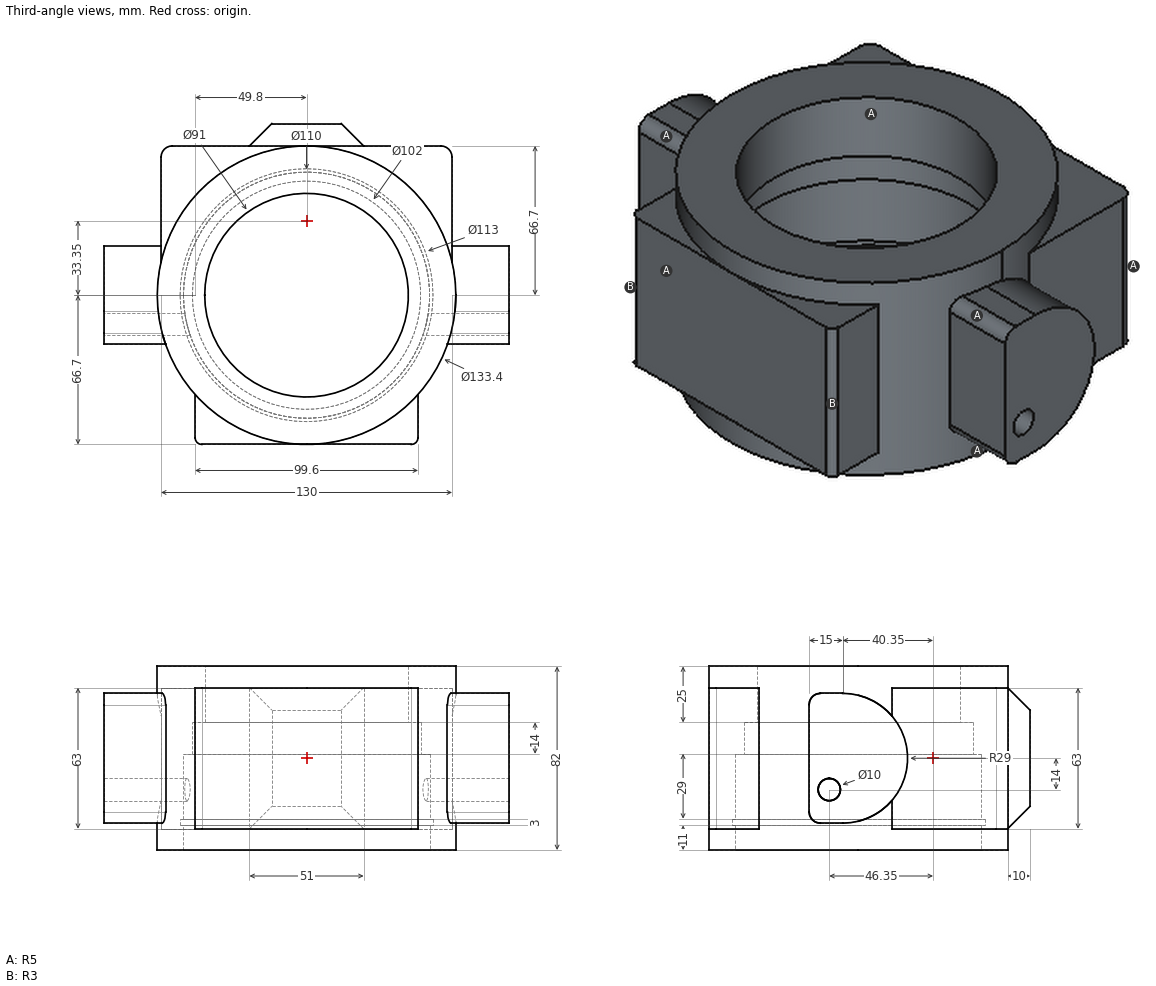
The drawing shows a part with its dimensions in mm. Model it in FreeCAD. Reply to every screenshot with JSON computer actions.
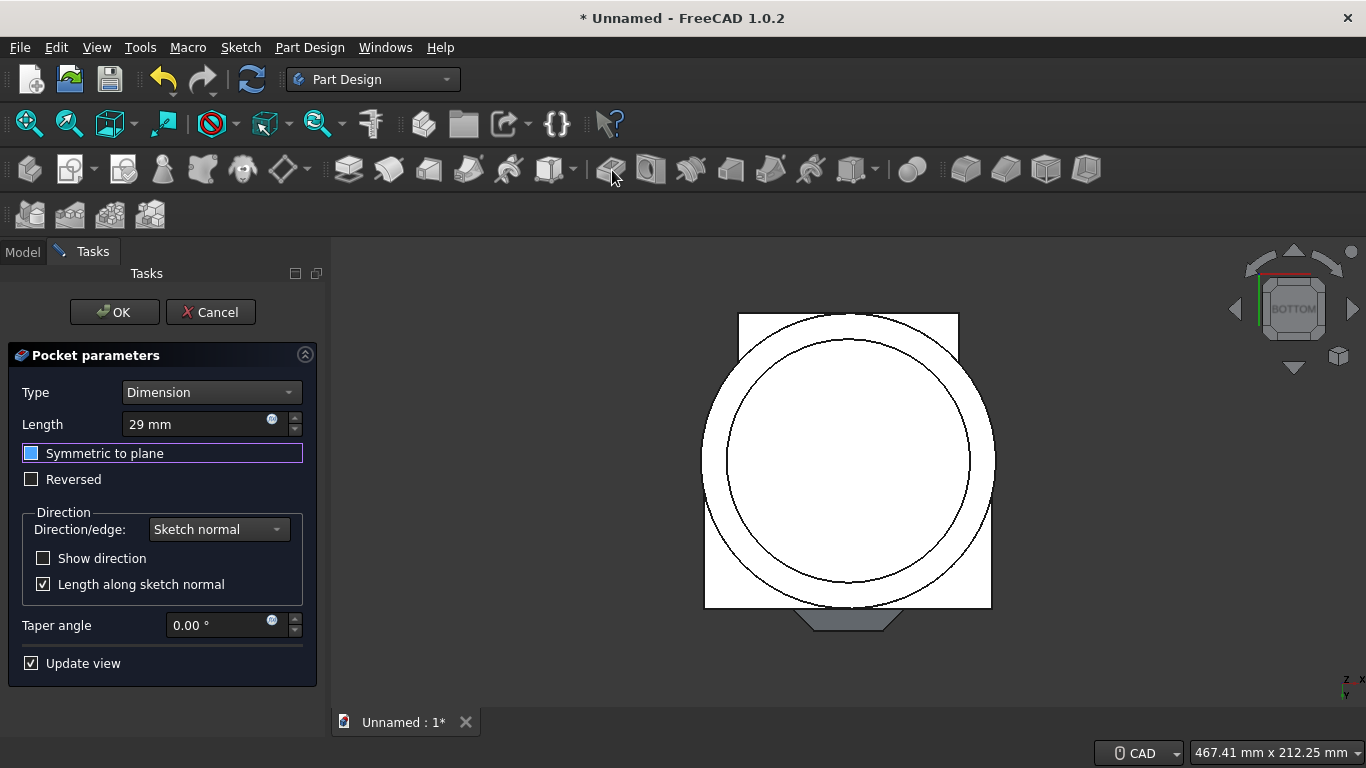
{"action": "left_click", "coordinate": [115, 312]}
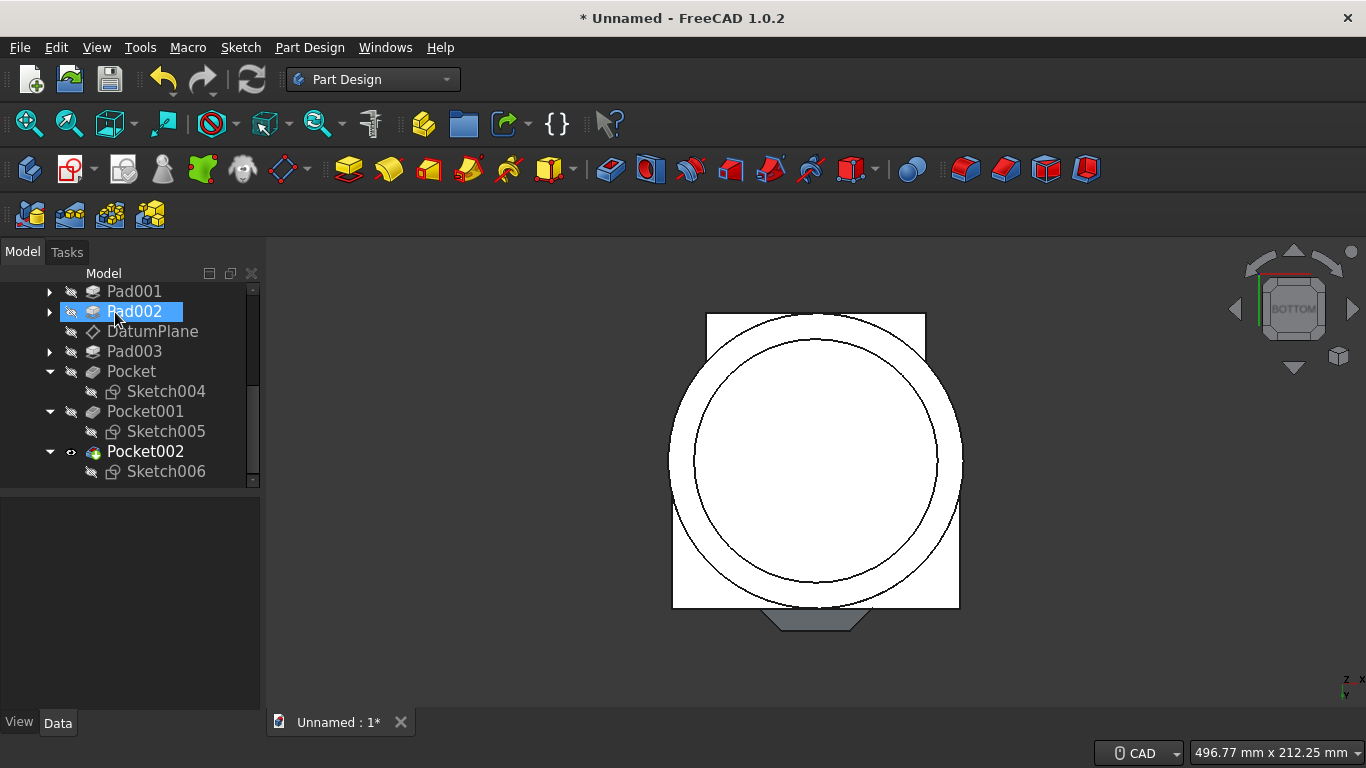
{"action": "left_click", "coordinate": [816, 460]}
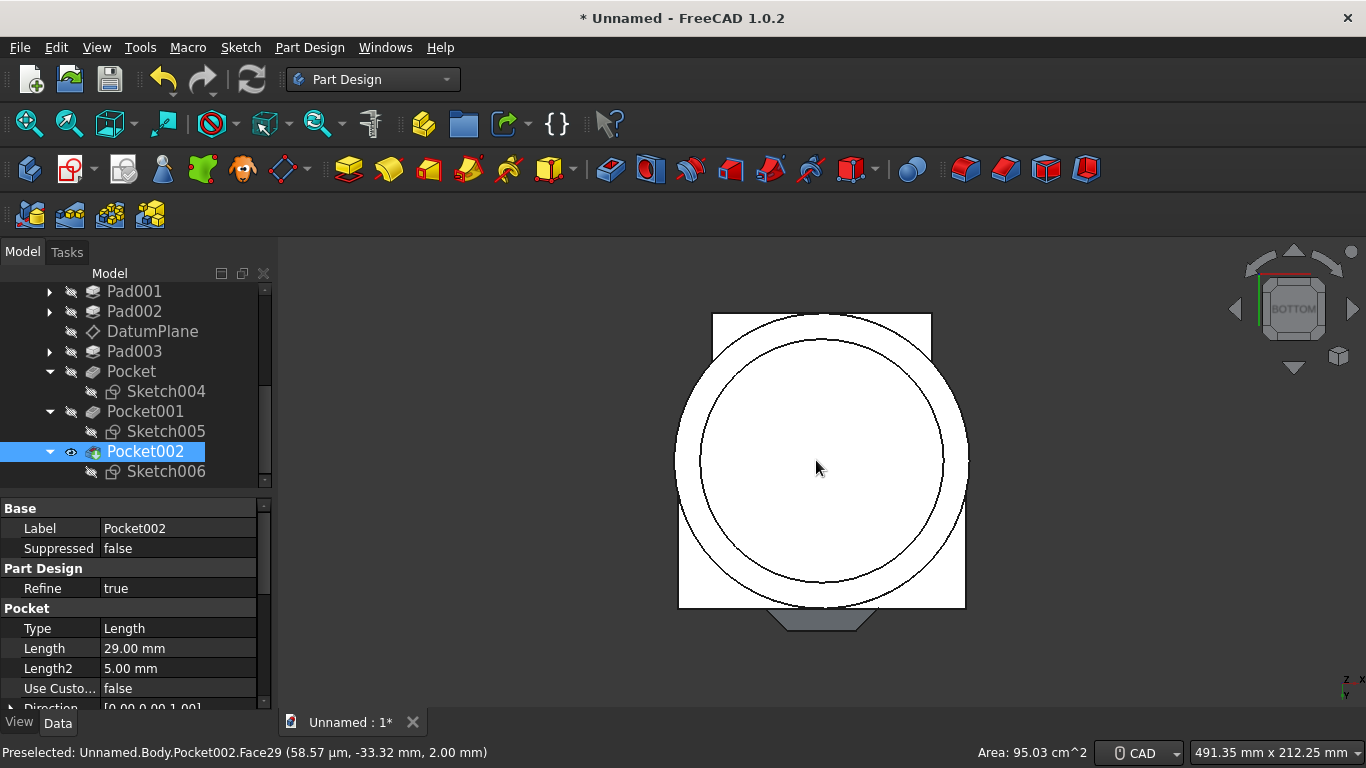
{"action": "left_click", "coordinate": [70, 170]}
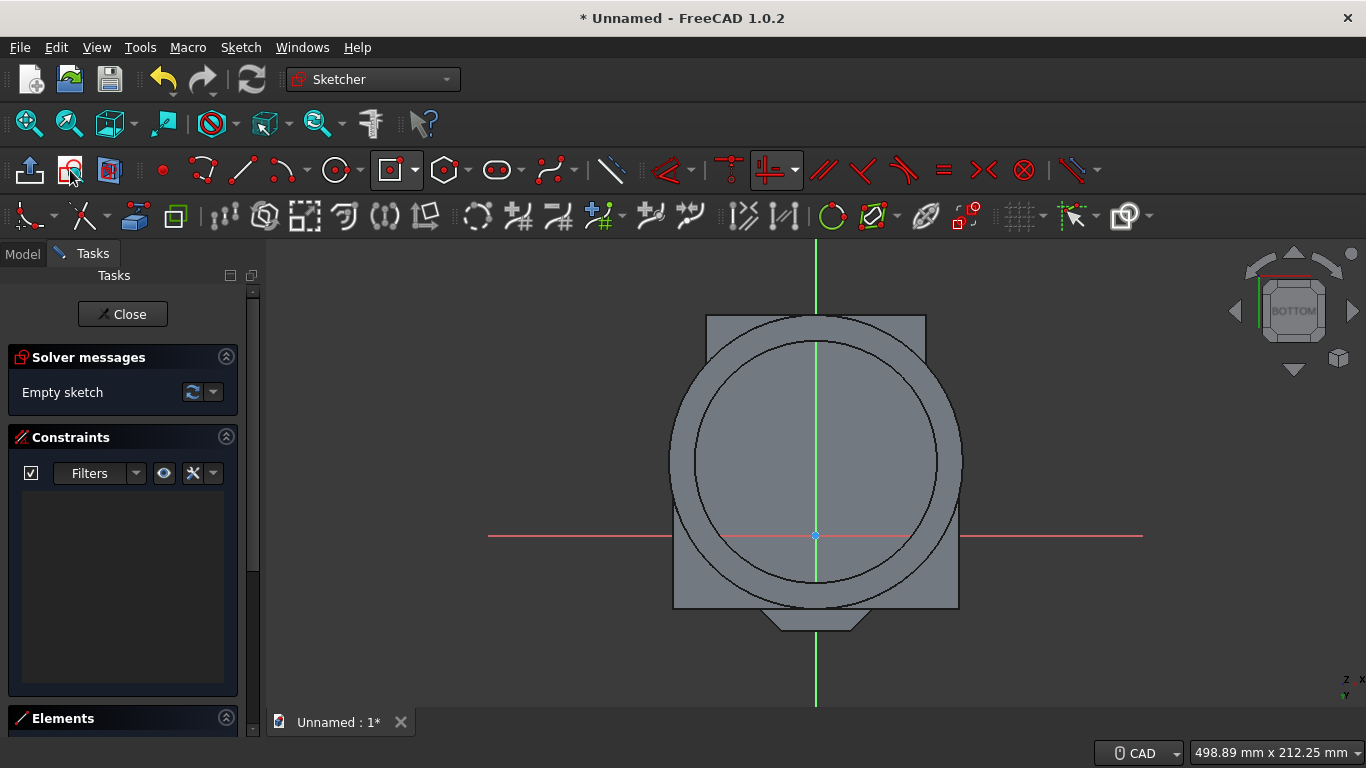
{"action": "key", "text": "q s"}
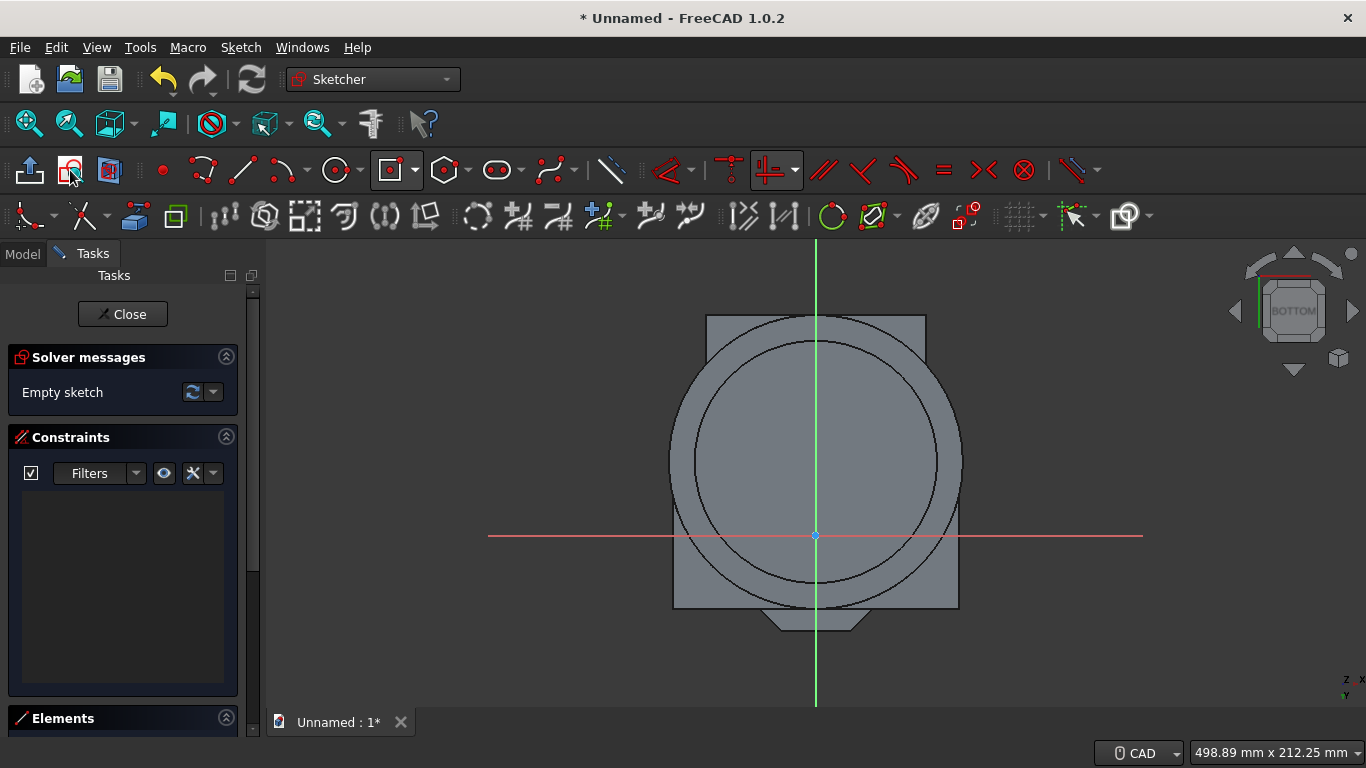
{"action": "key", "text": "g c"}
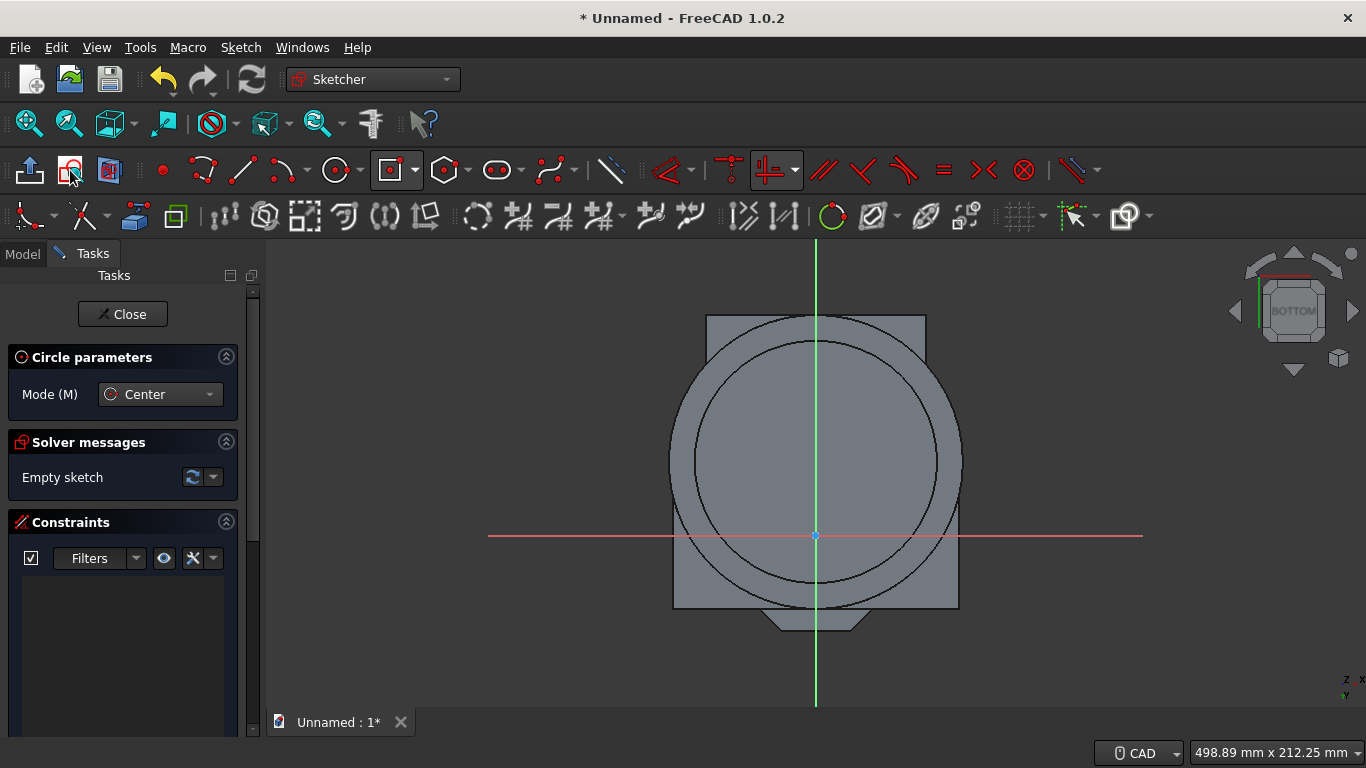
{"action": "left_click", "coordinate": [816, 462]}
{"action": "left_click", "coordinate": [895, 382]}
{"action": "key", "text": "Escape"}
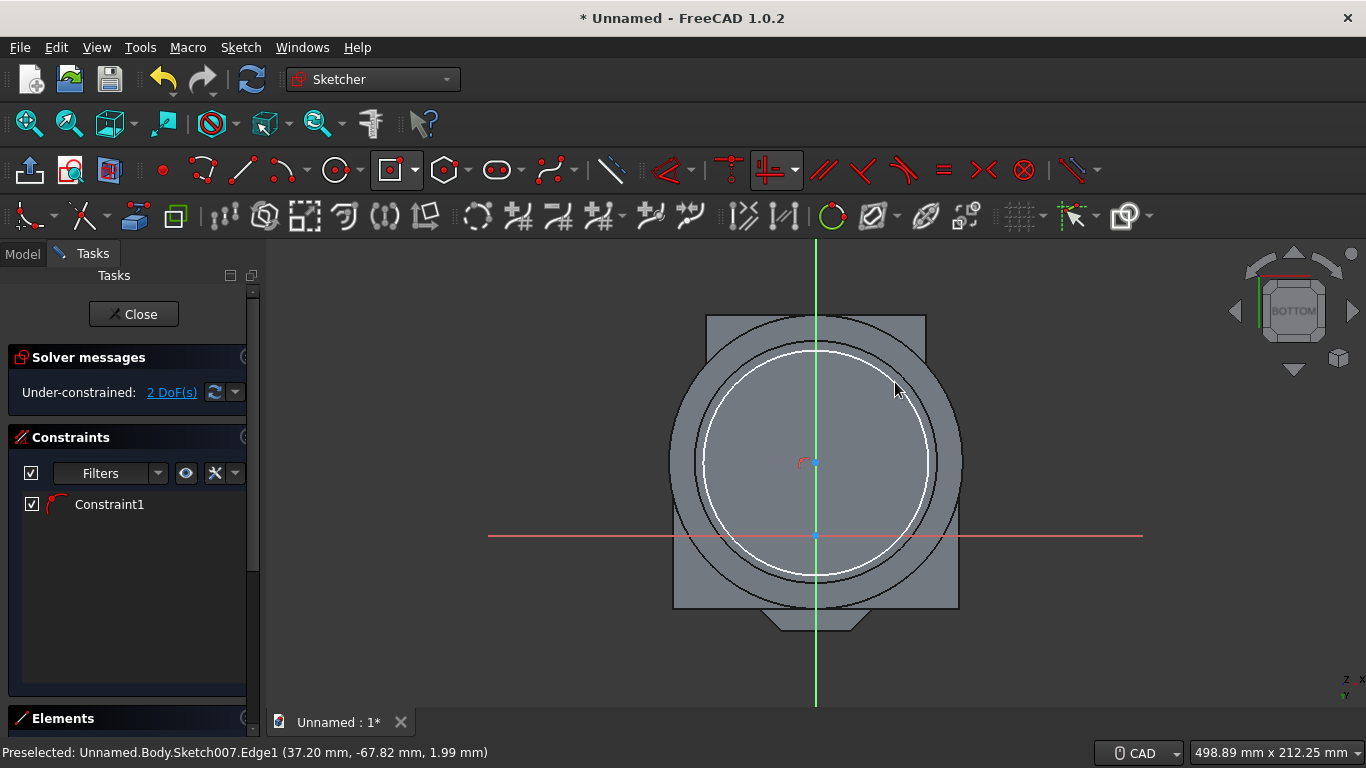
{"action": "key", "text": "d"}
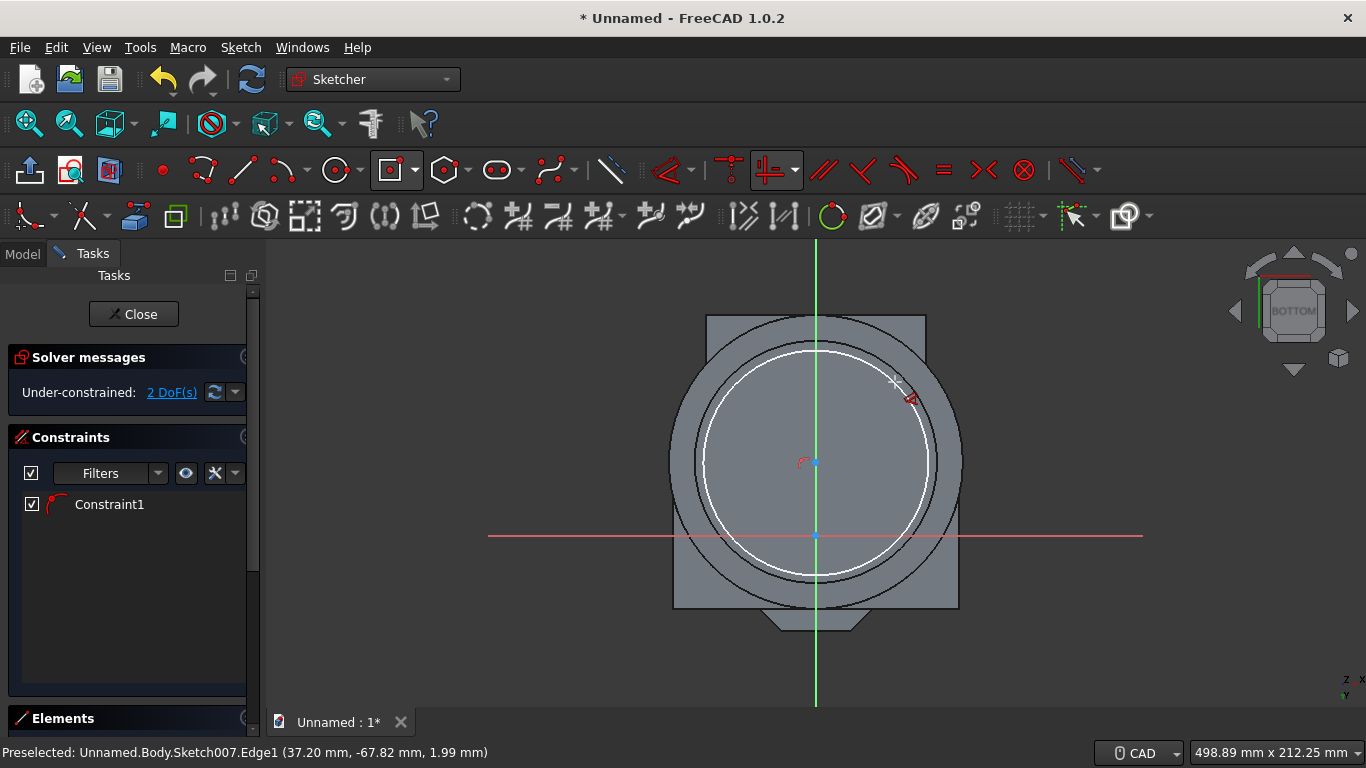
{"action": "left_click", "coordinate": [895, 383]}
{"action": "left_click", "coordinate": [918, 360]}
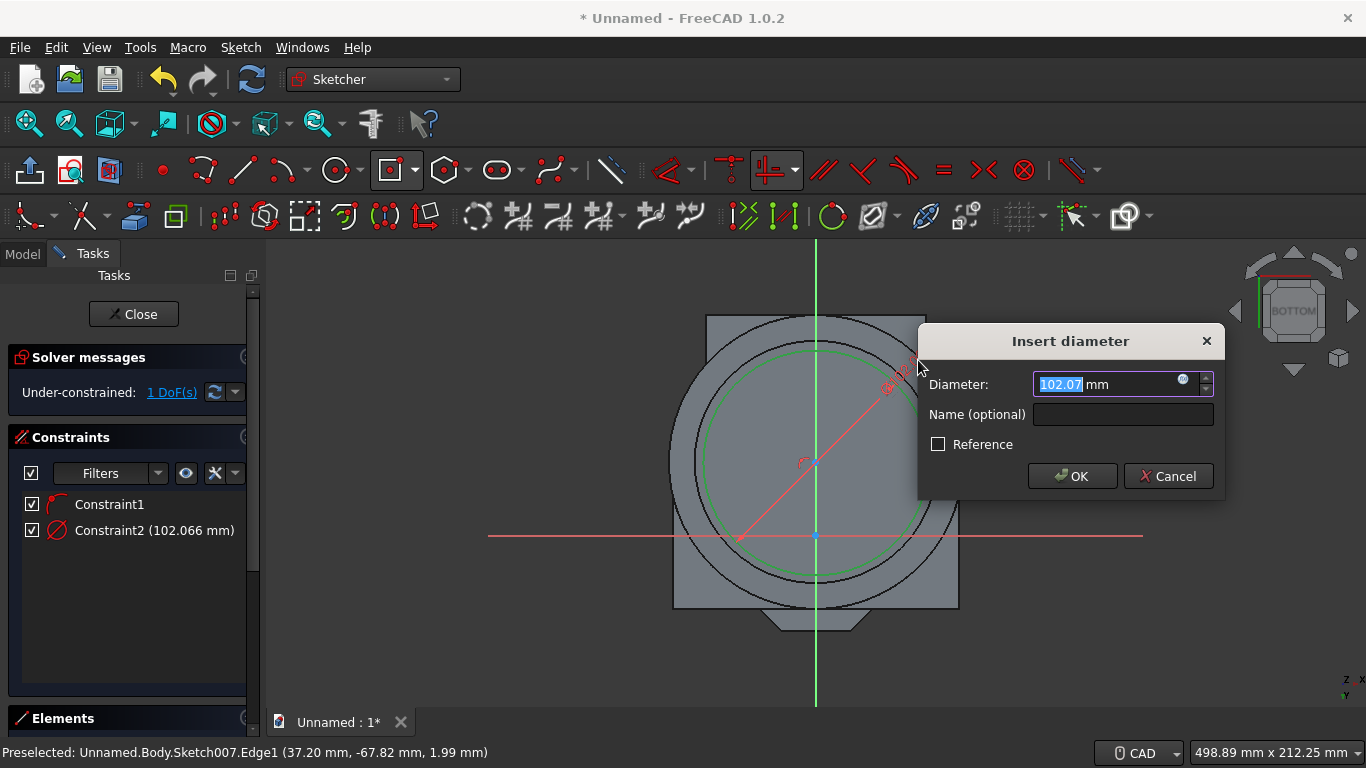
{"action": "type", "text": "102"}
{"action": "key", "text": "Return"}